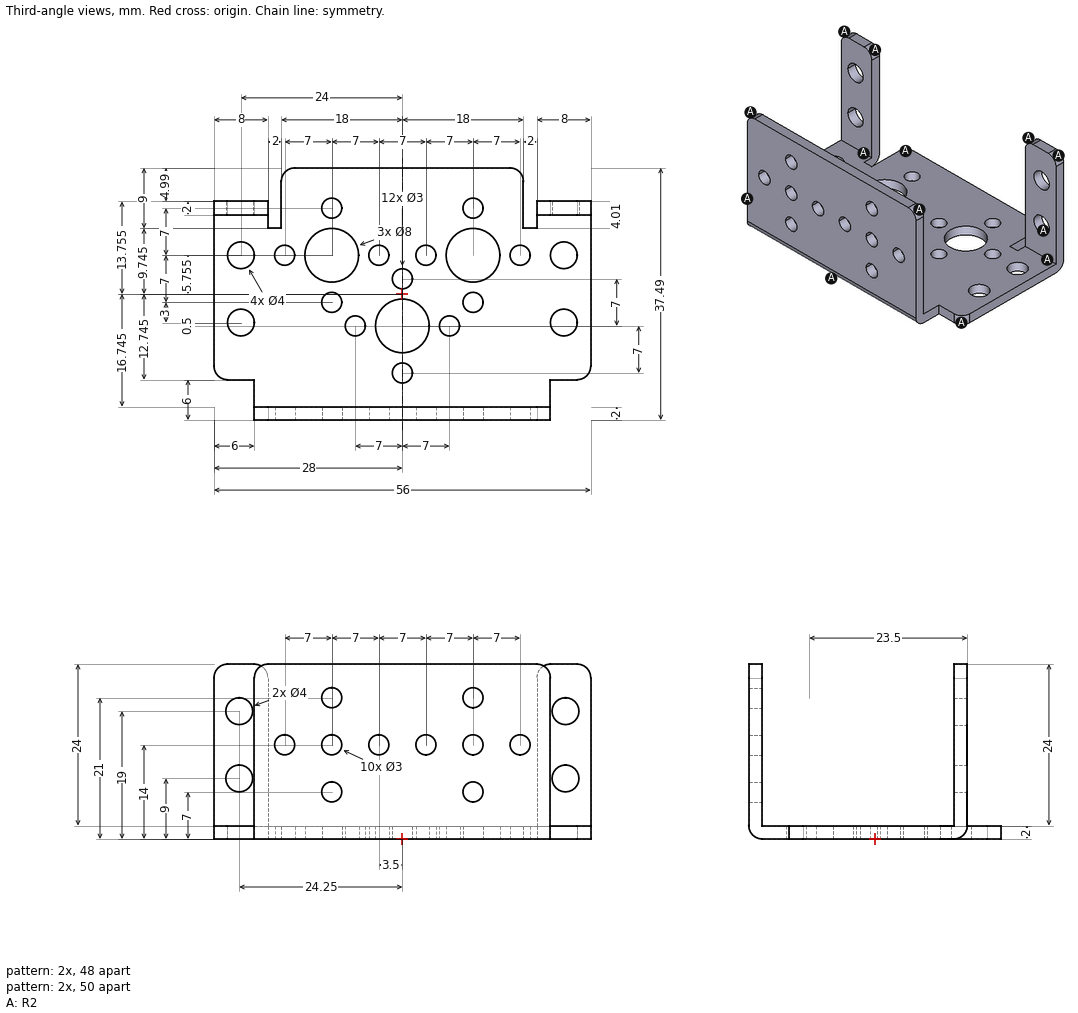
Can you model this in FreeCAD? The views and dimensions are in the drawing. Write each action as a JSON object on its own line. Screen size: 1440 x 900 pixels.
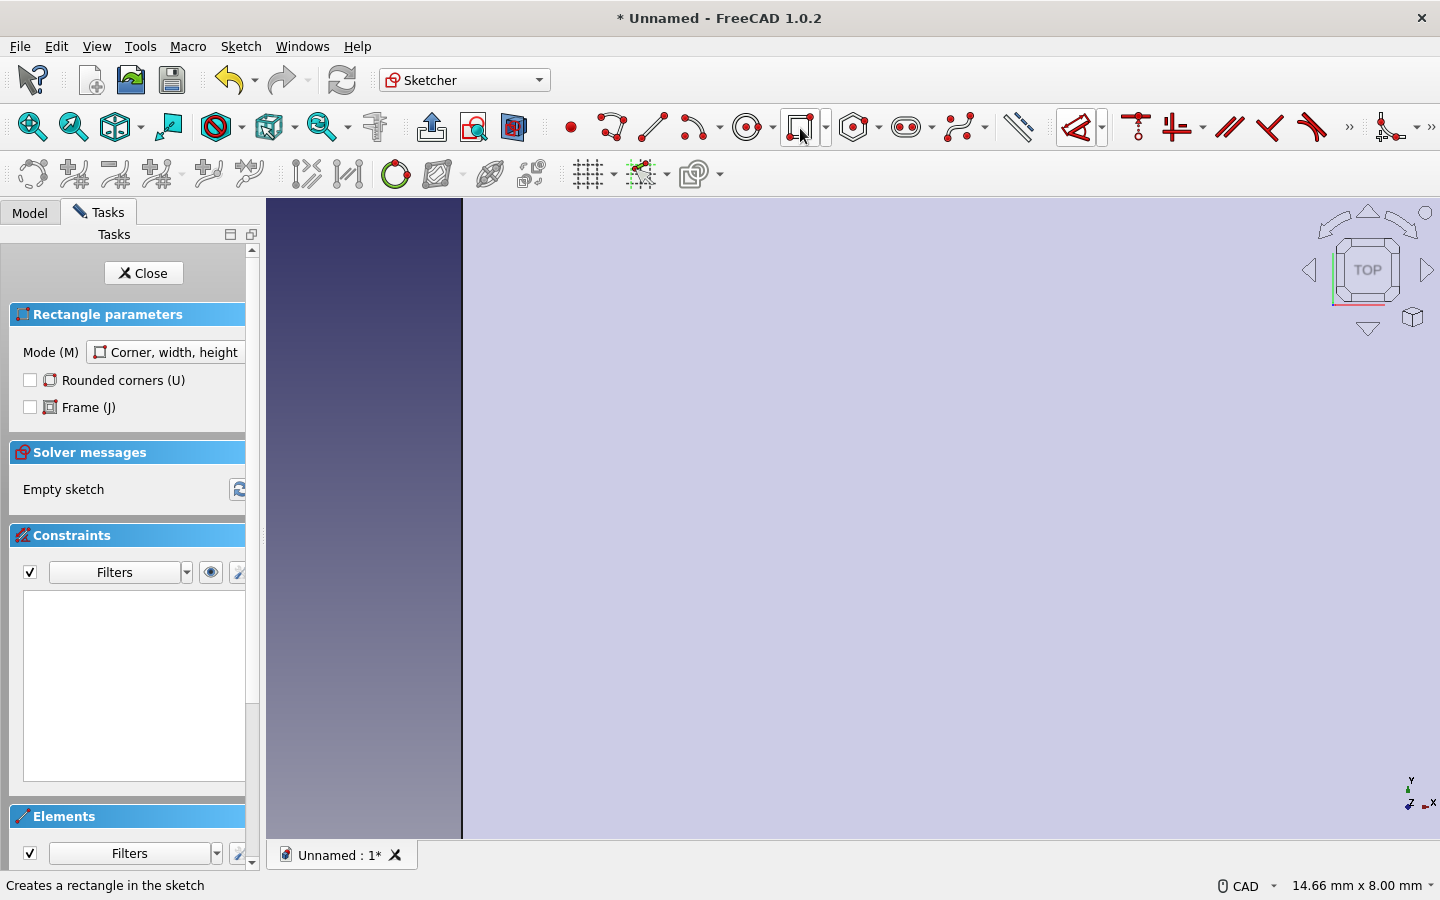
{"action": "left_click", "coordinate": [462, 438]}
{"action": "mouse_move", "coordinate": [1103, 598]}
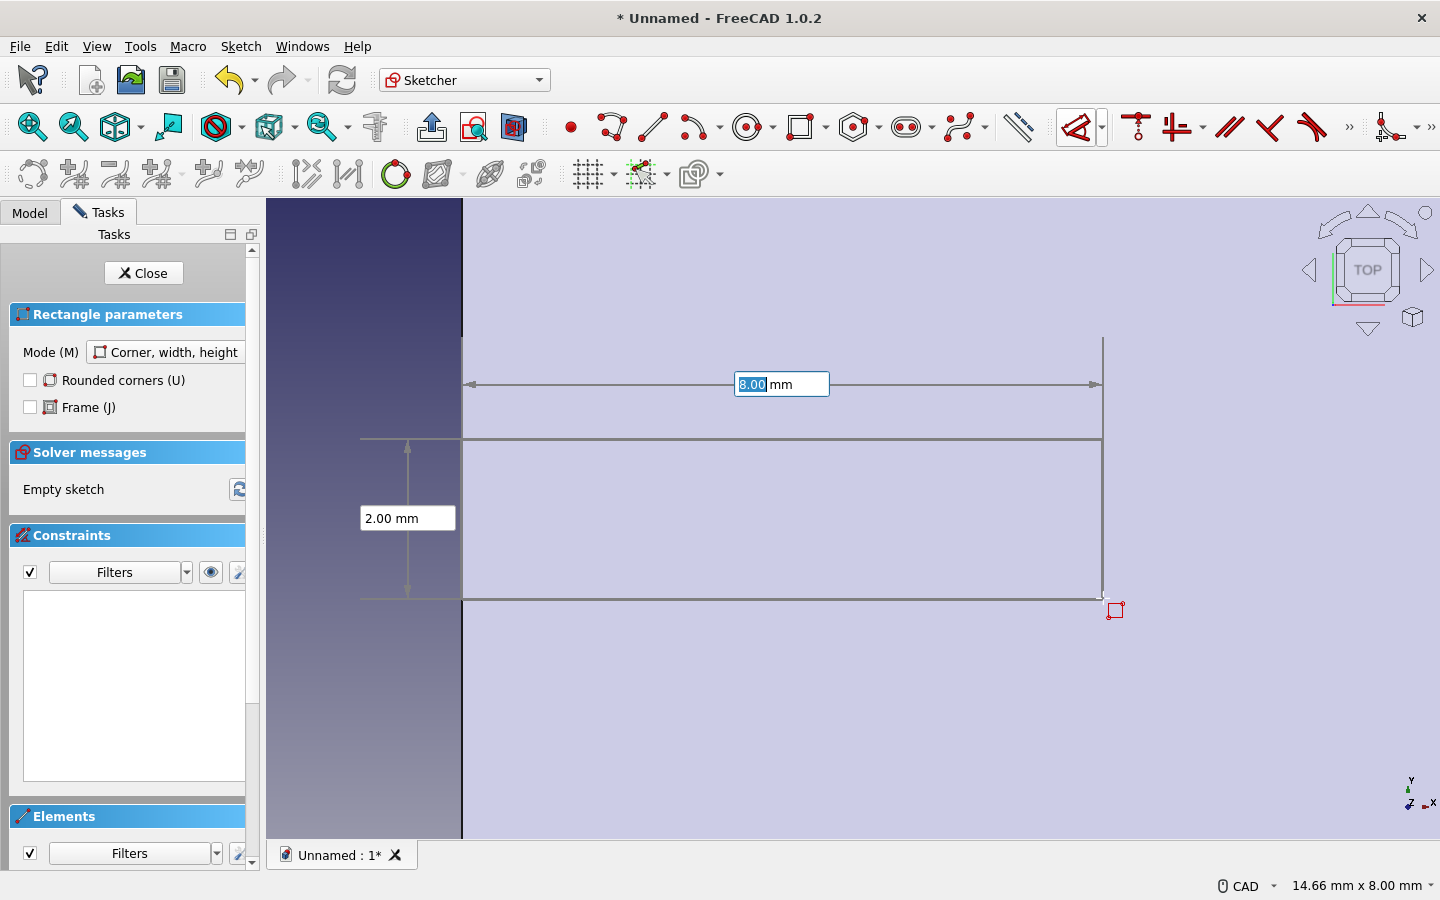
{"action": "type", "text": "8"}
{"action": "key", "text": "Tab"}
{"action": "type", "text": "2"}
{"action": "key", "text": "Return"}
{"action": "key", "text": "Escape"}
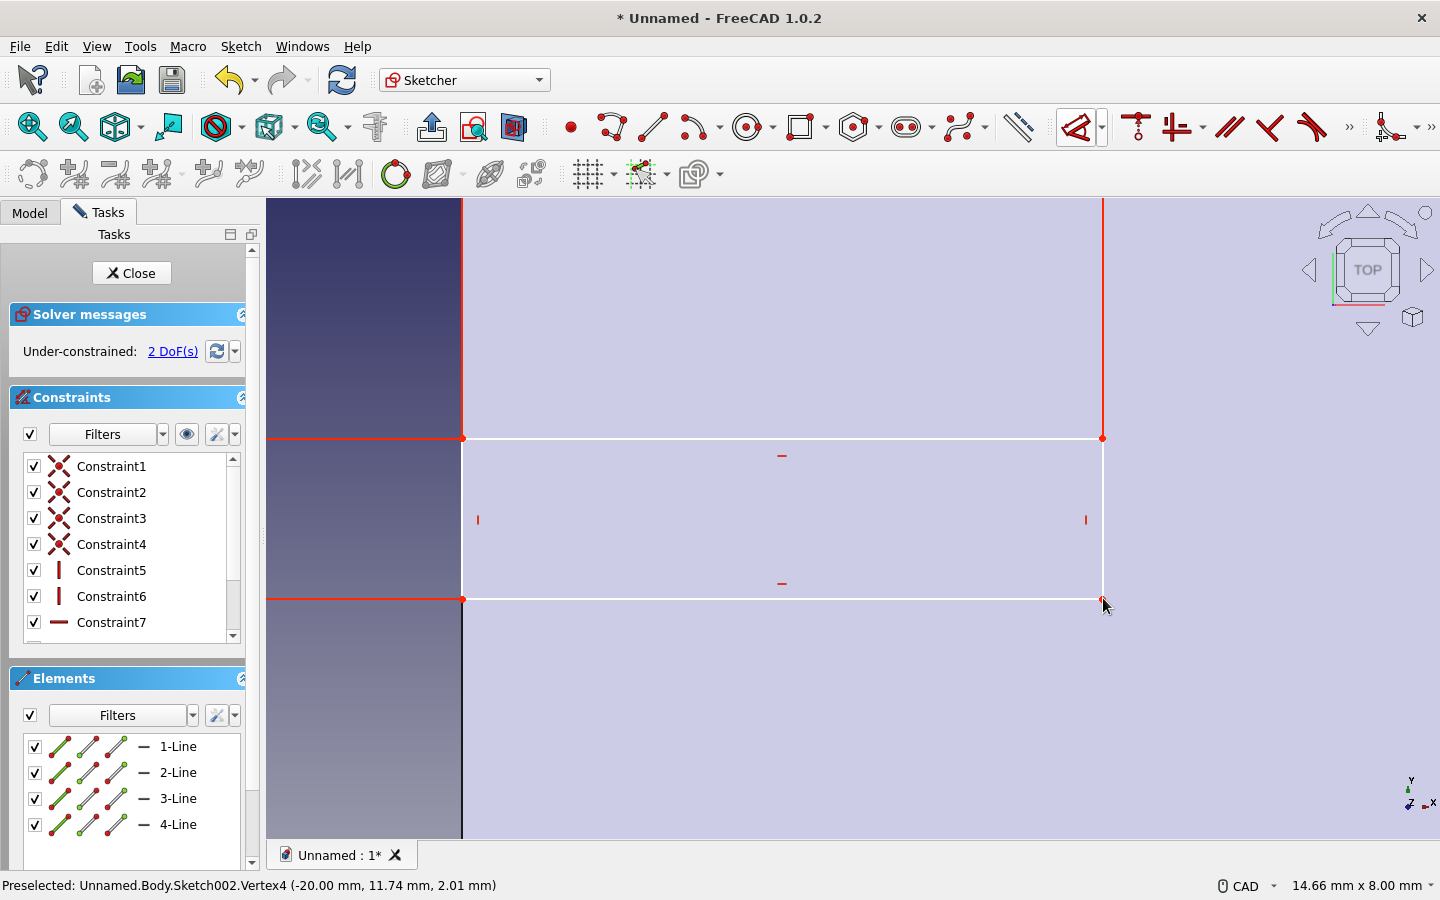
{"action": "left_click", "coordinate": [462, 439]}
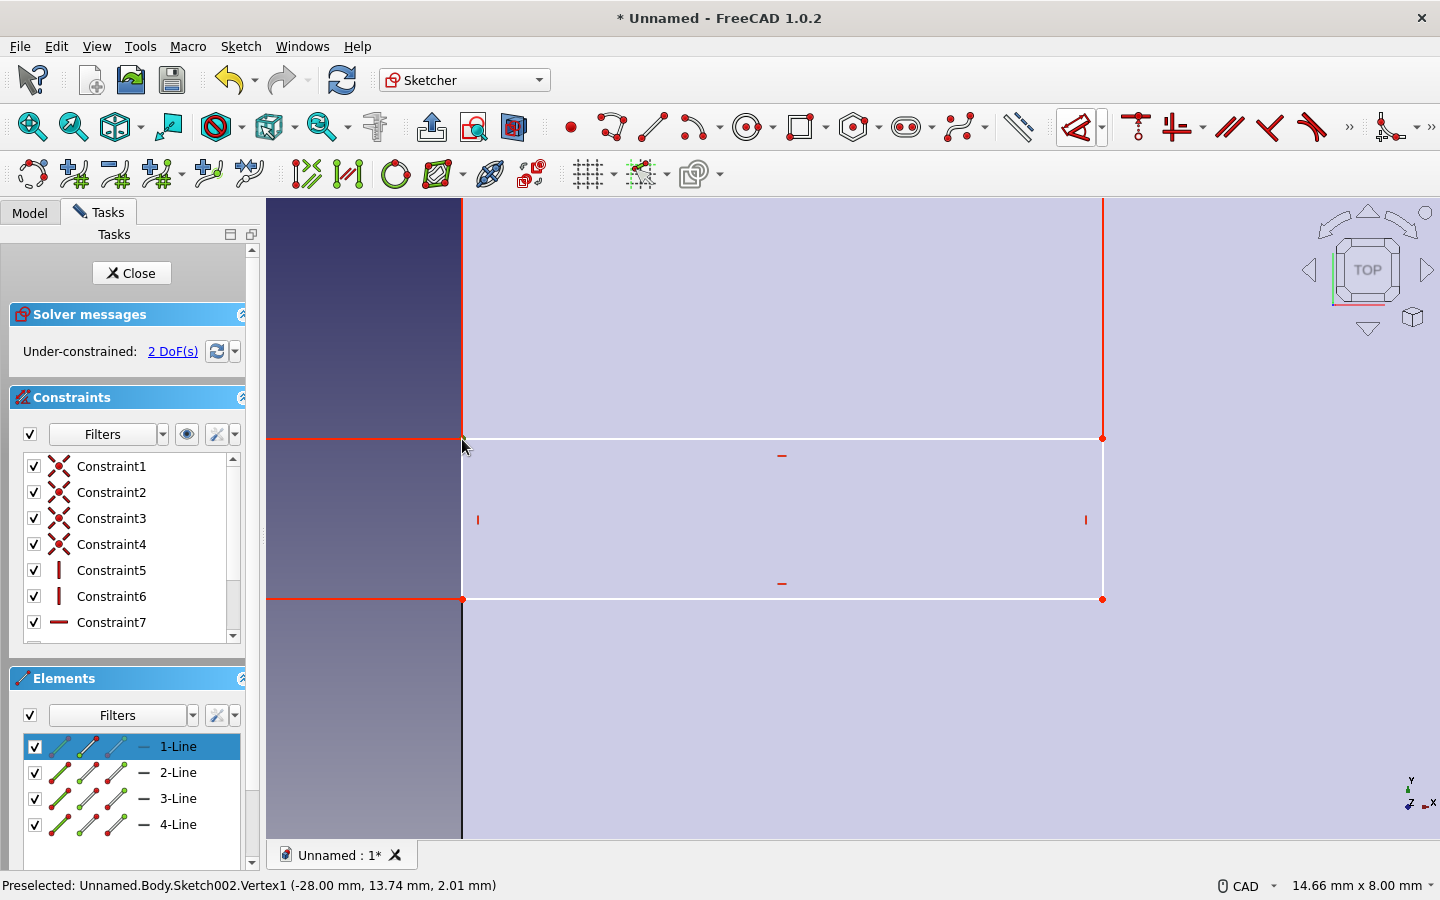
{"action": "key", "text": "l"}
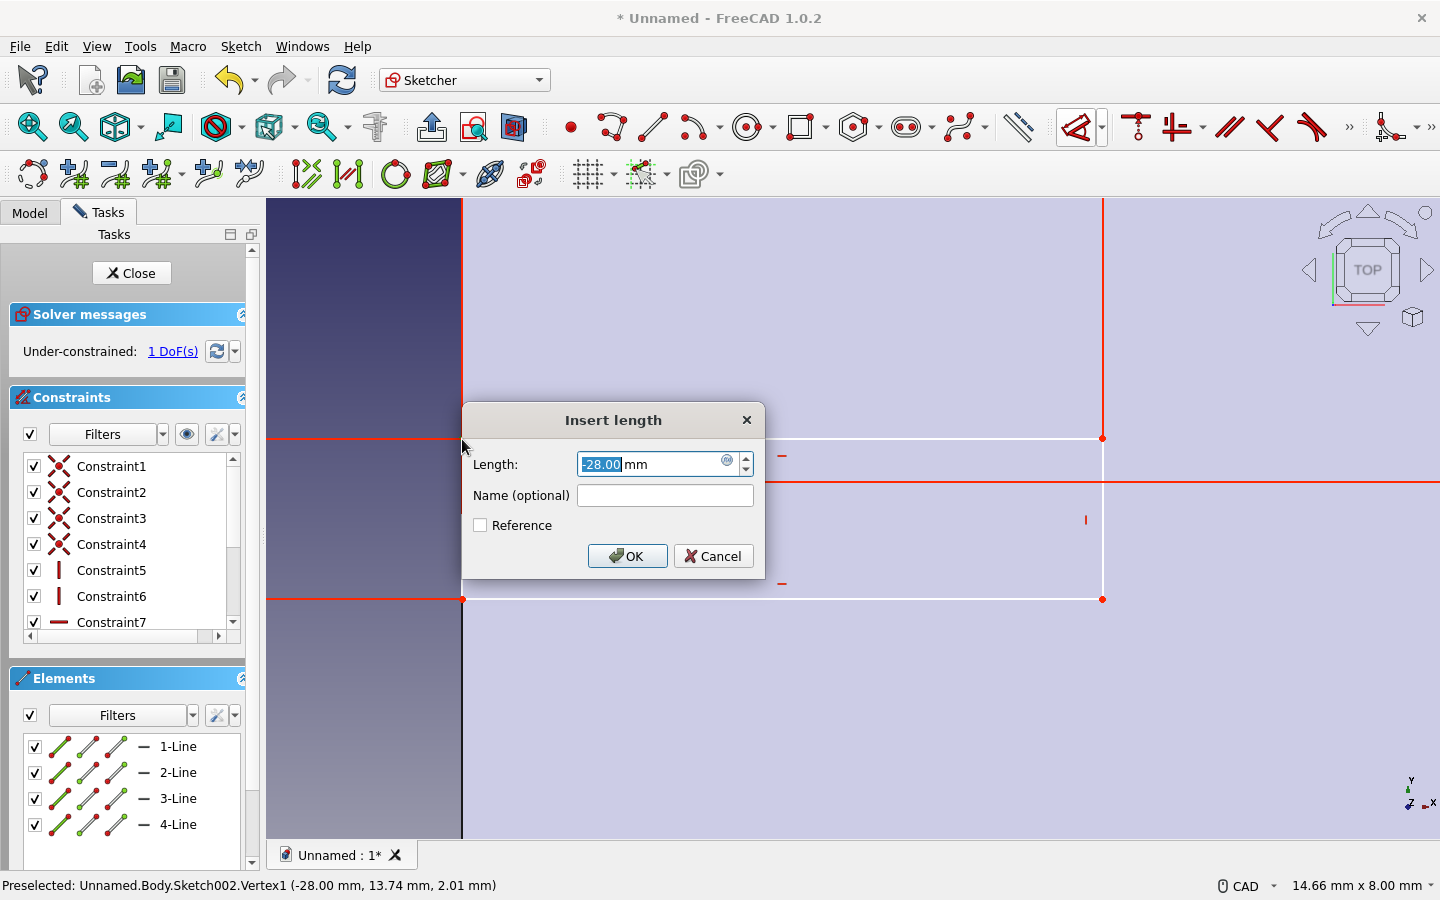
{"action": "type", "text": "-28"}
{"action": "key", "text": "Return"}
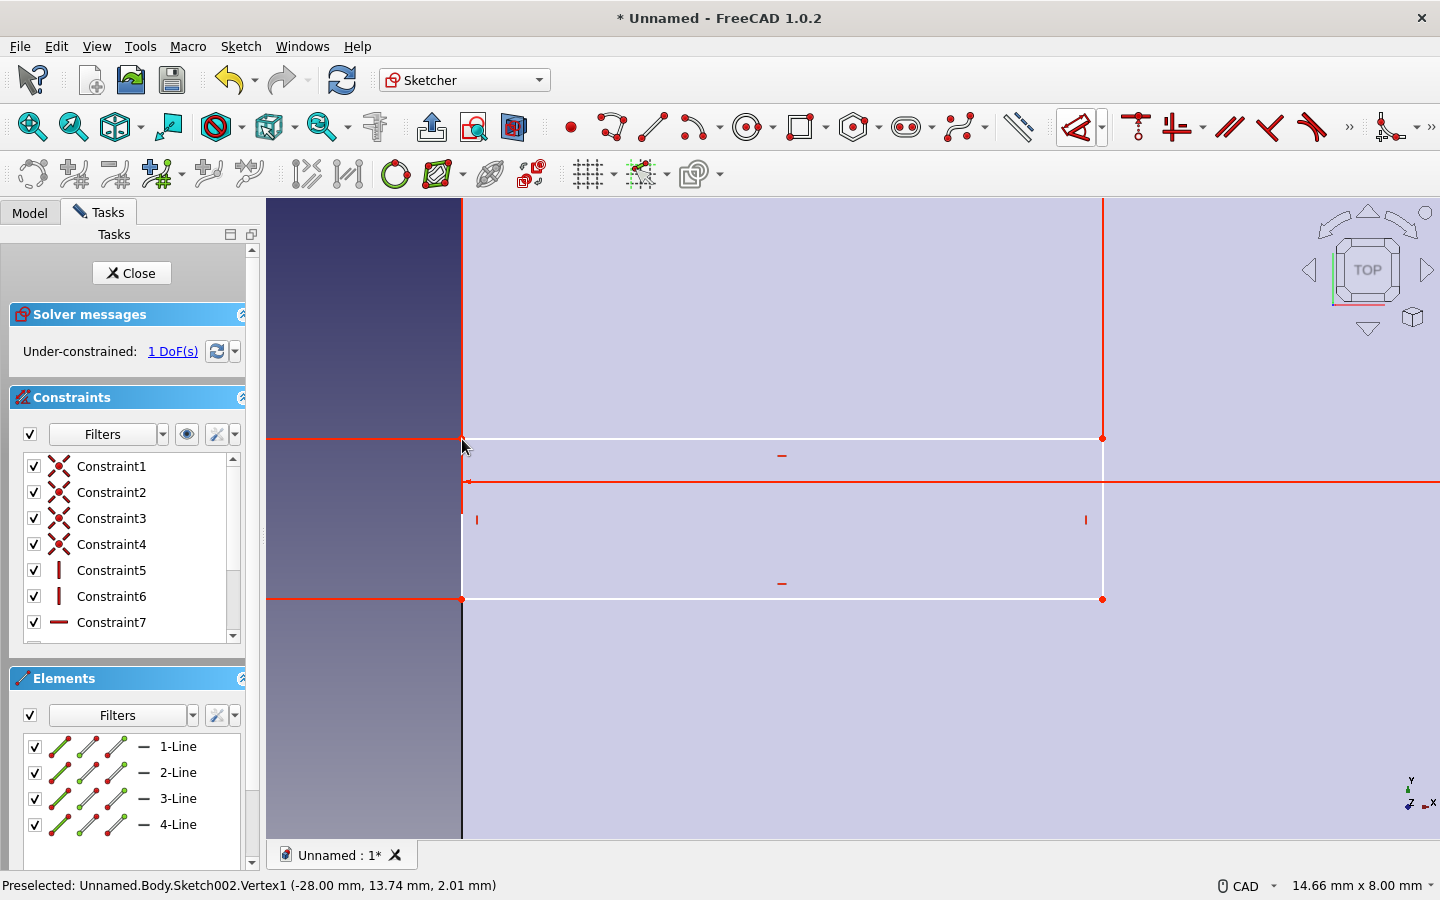
{"action": "left_click", "coordinate": [462, 439]}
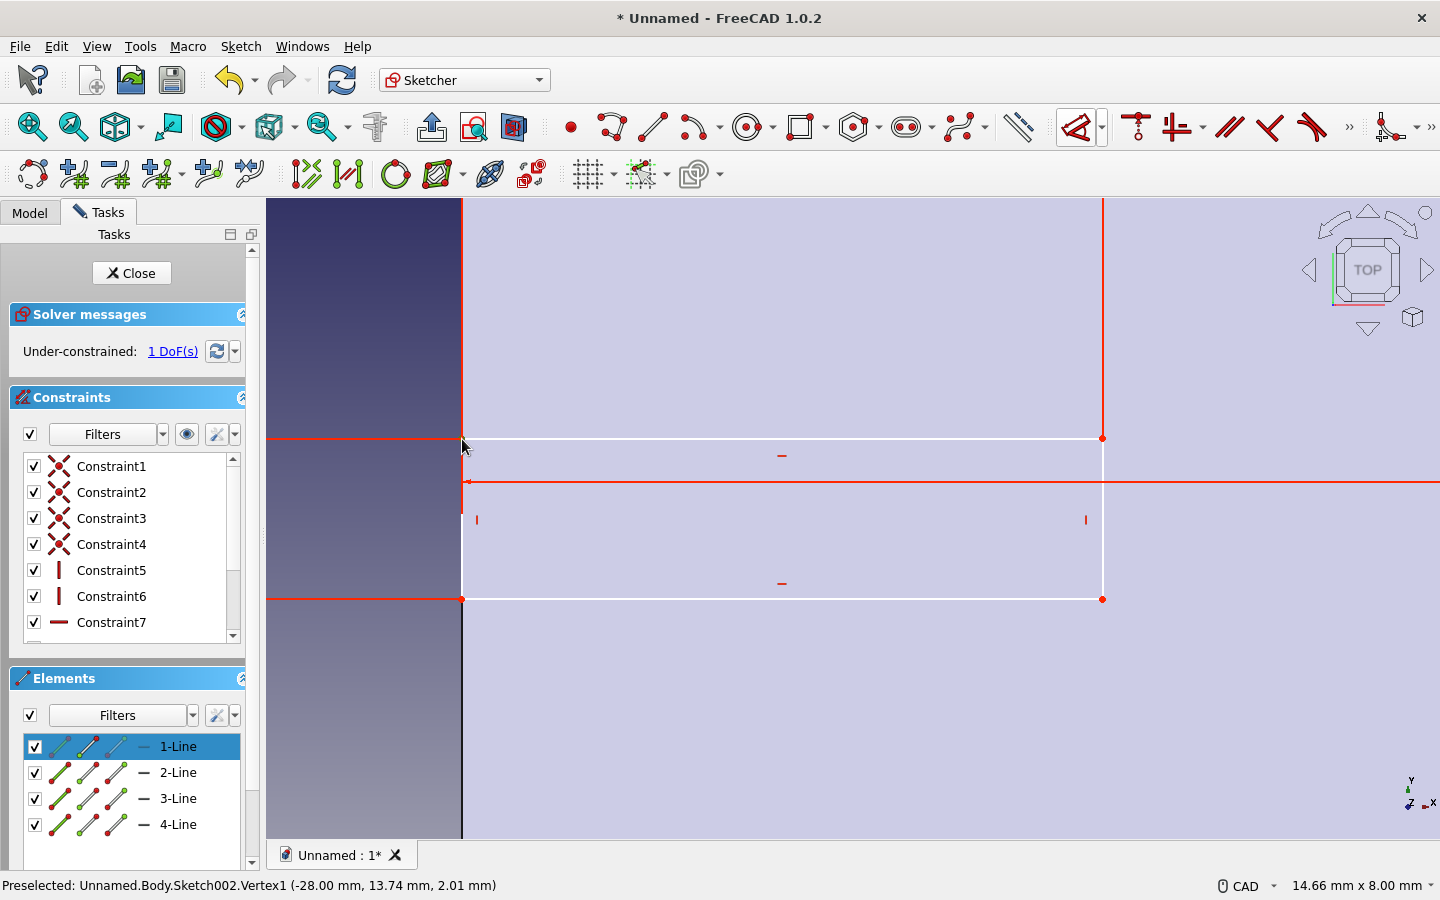
{"action": "key", "text": "i"}